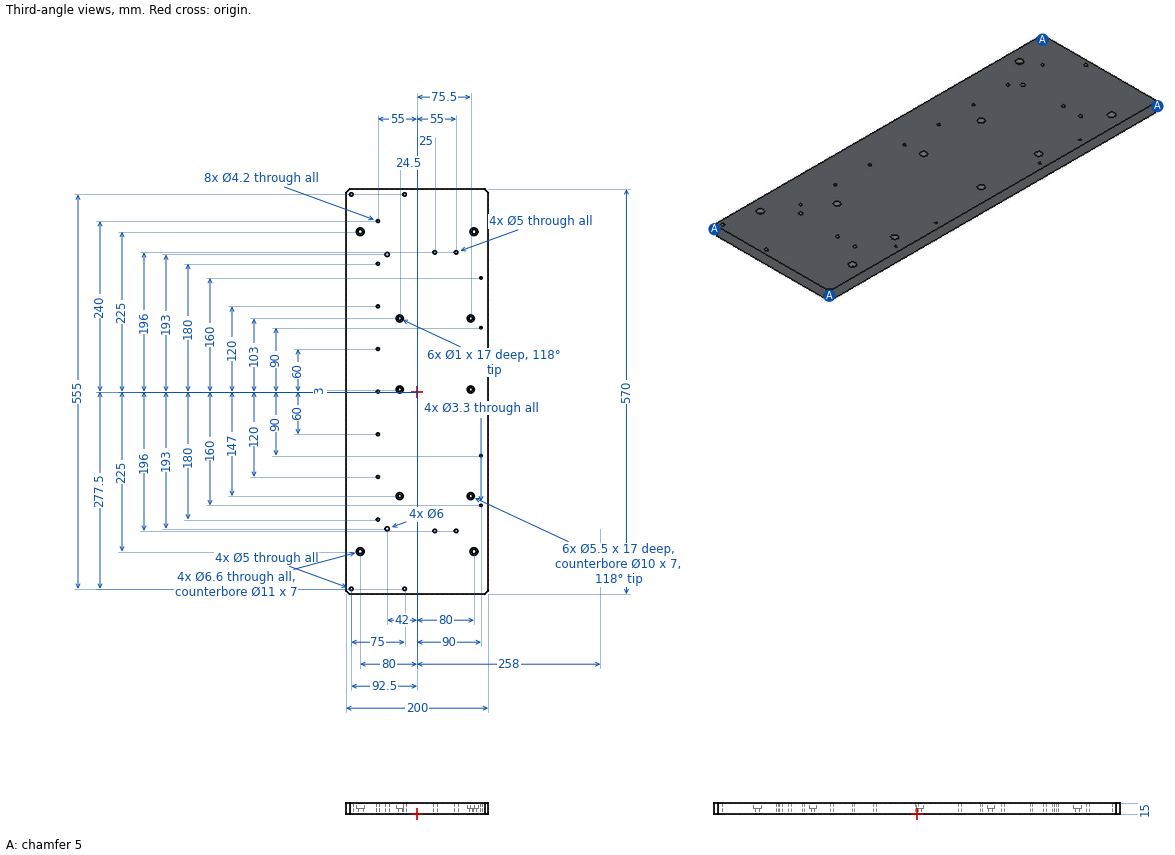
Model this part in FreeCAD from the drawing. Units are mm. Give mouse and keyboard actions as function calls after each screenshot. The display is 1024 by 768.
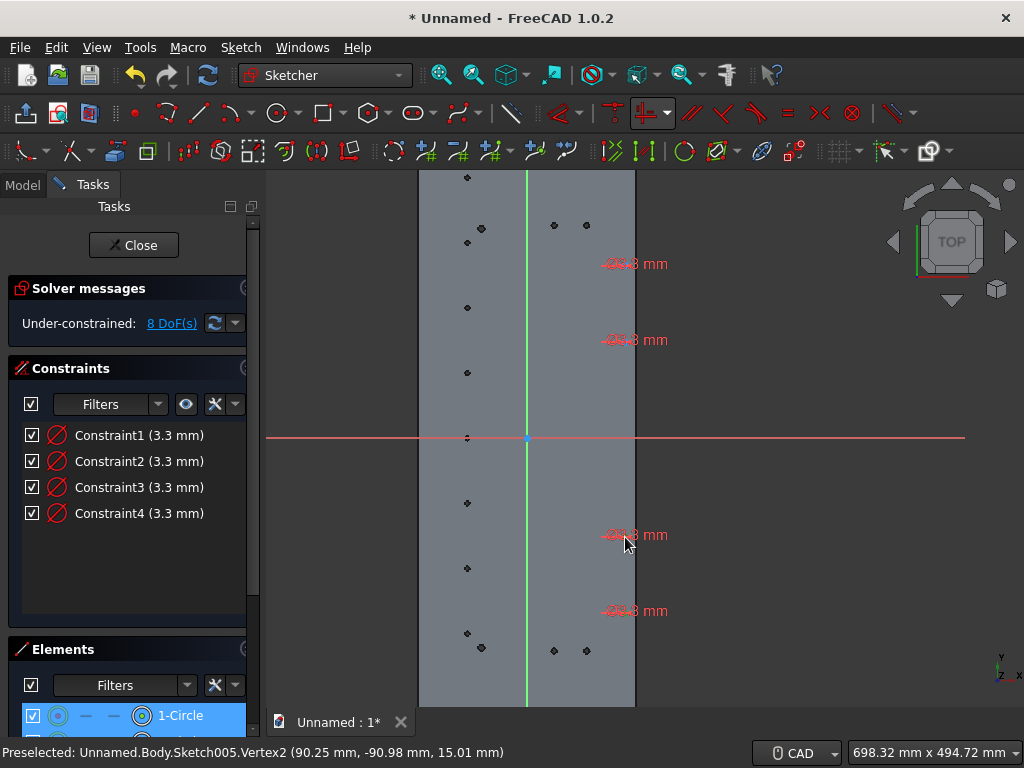
key(v)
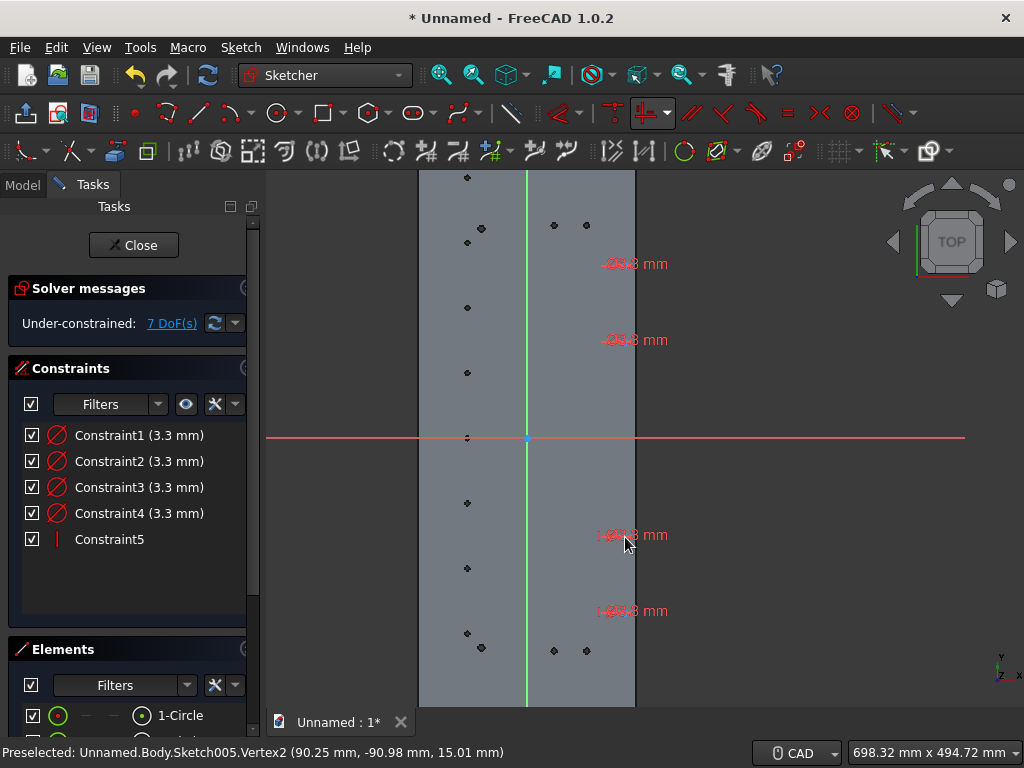
click(625, 537)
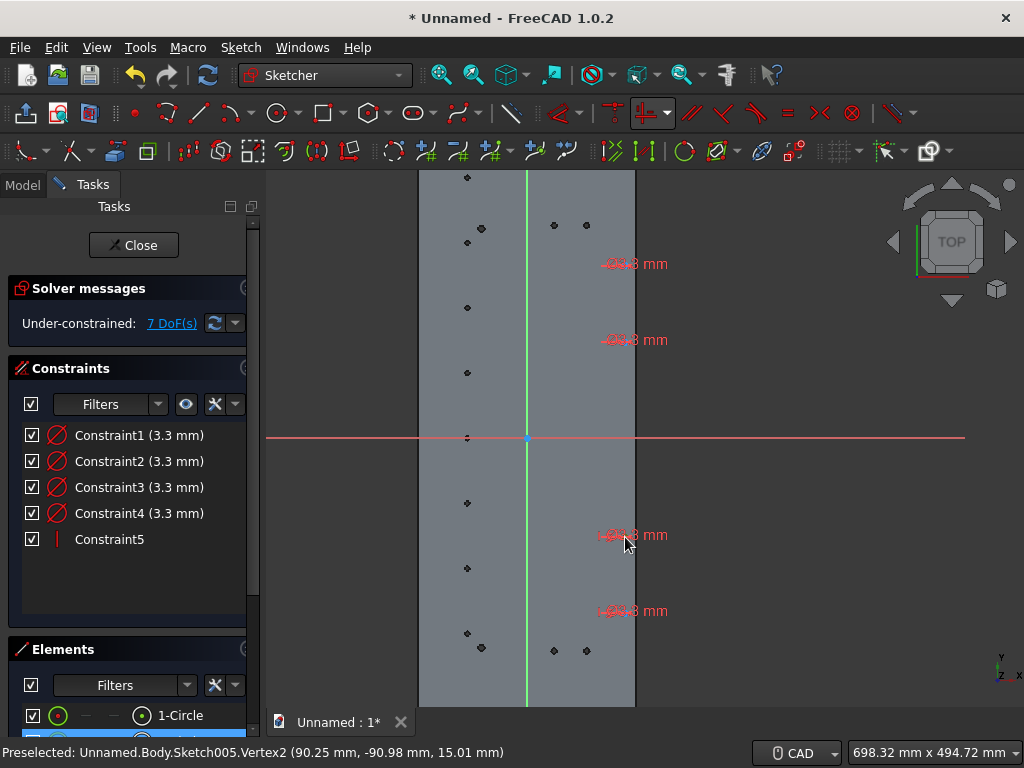
click(625, 342)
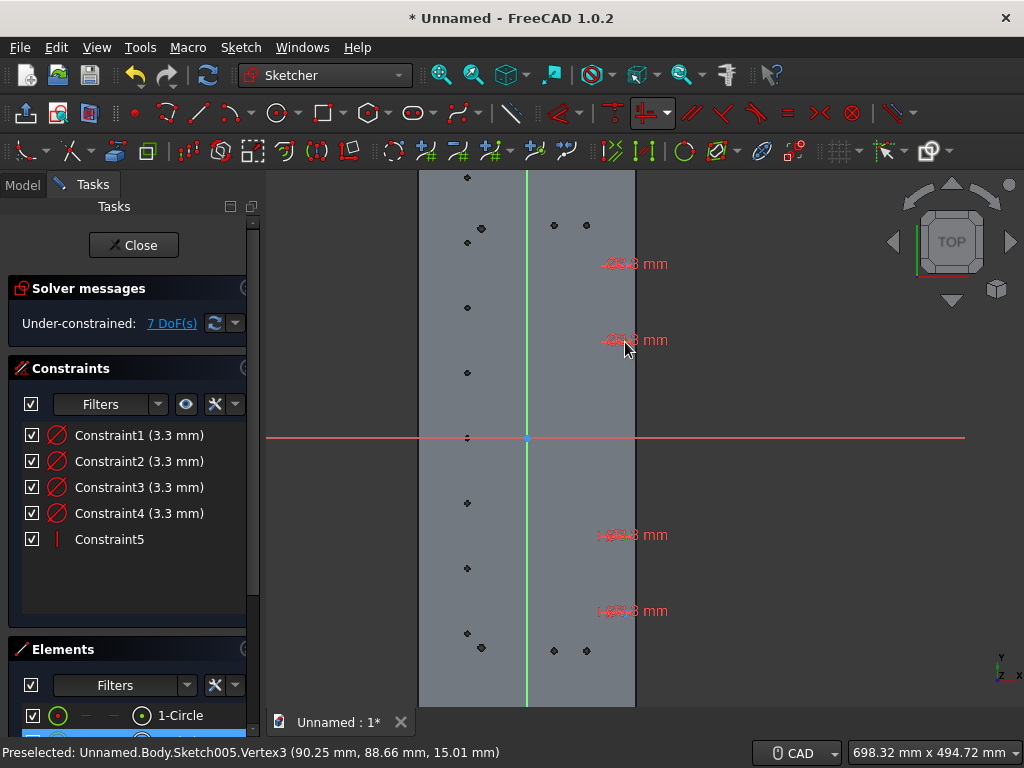
click(670, 114)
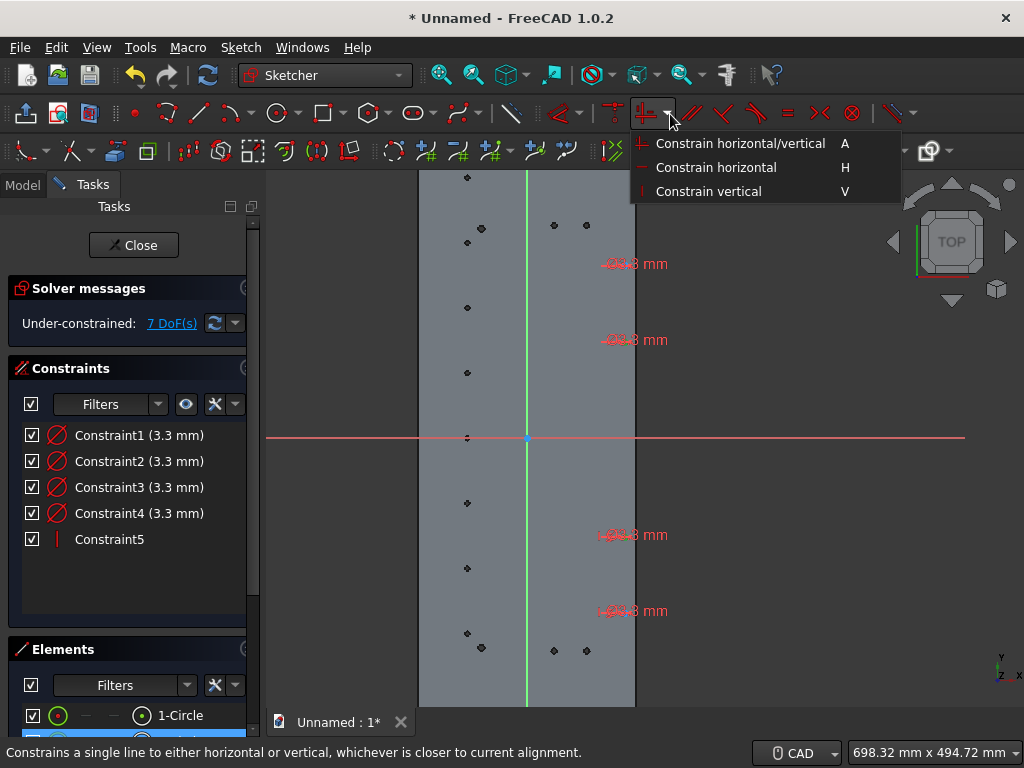
click(766, 191)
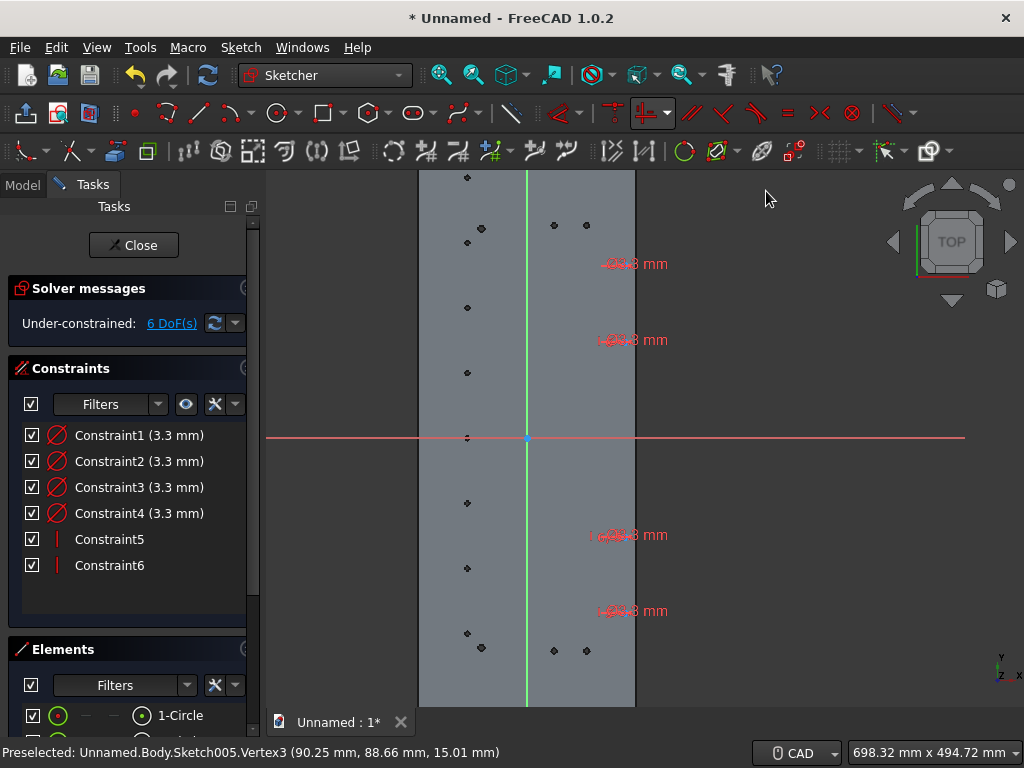
click(625, 342)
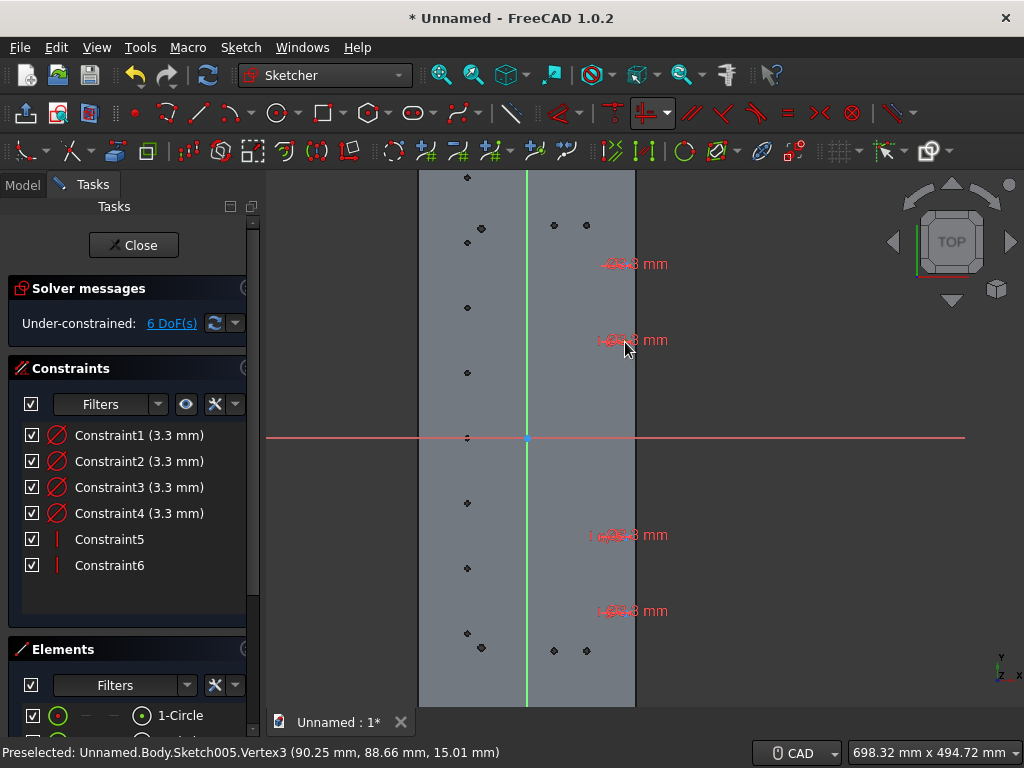
click(625, 266)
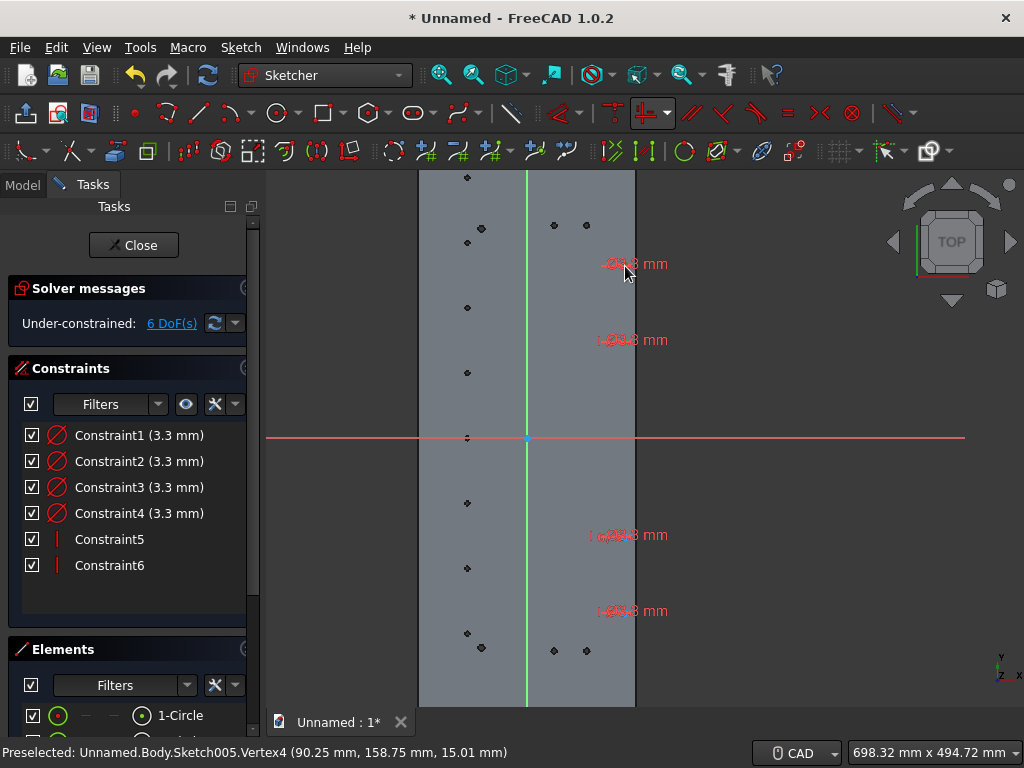
click(670, 114)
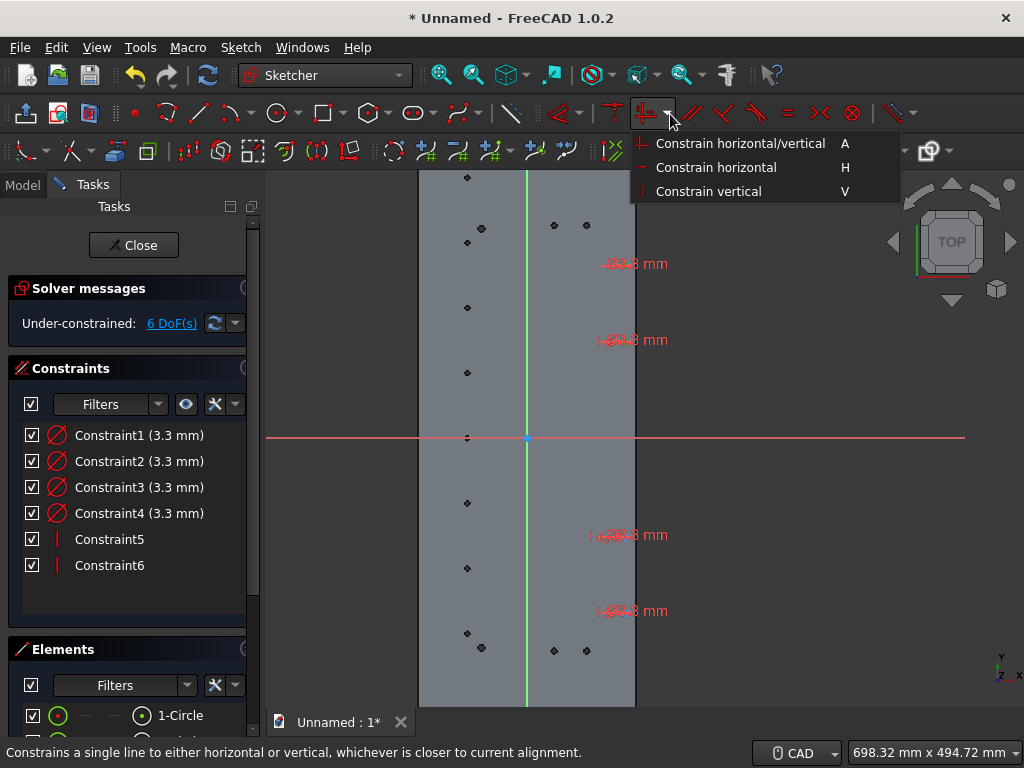
click(766, 191)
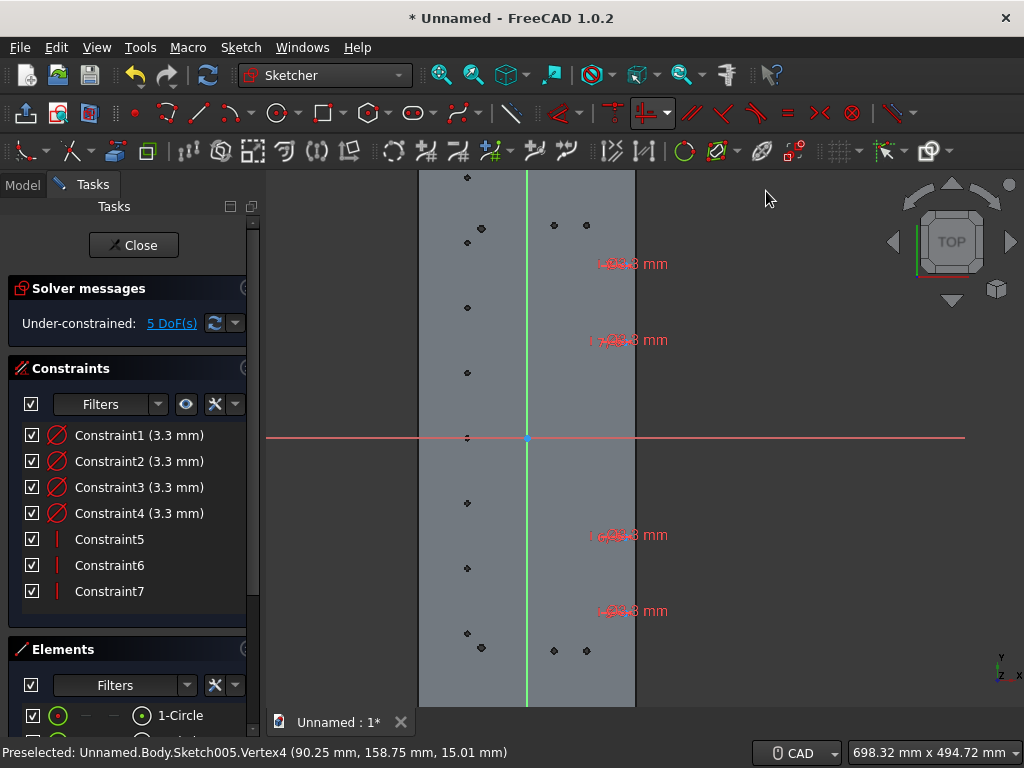
click(558, 114)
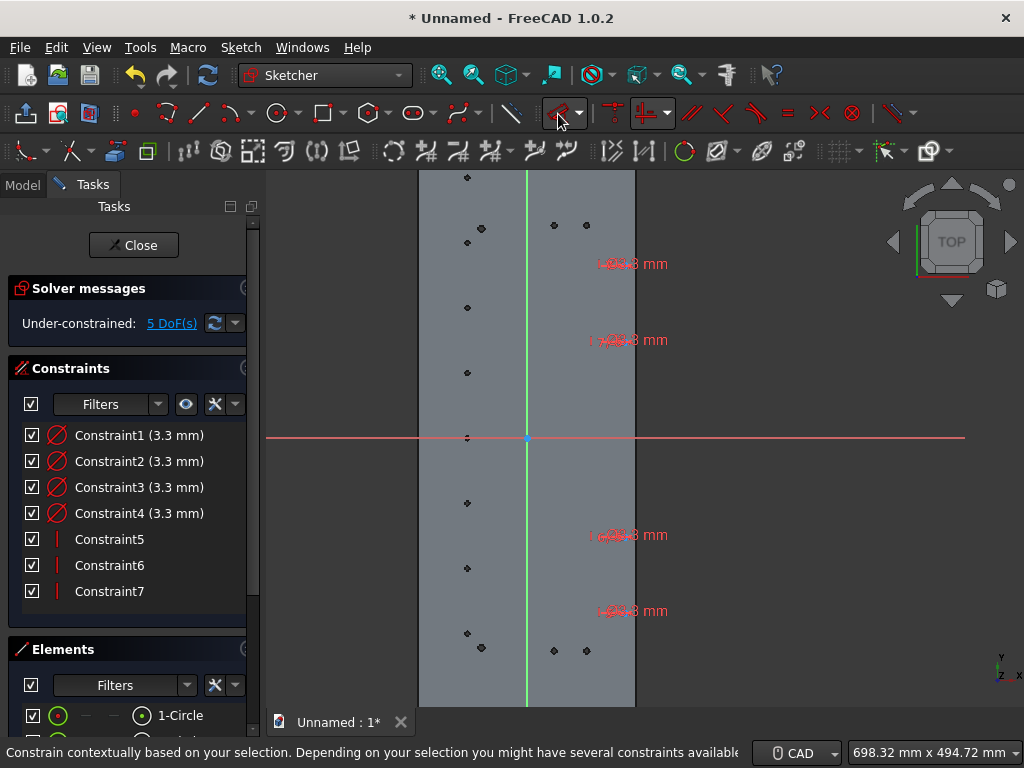
click(625, 613)
click(576, 647)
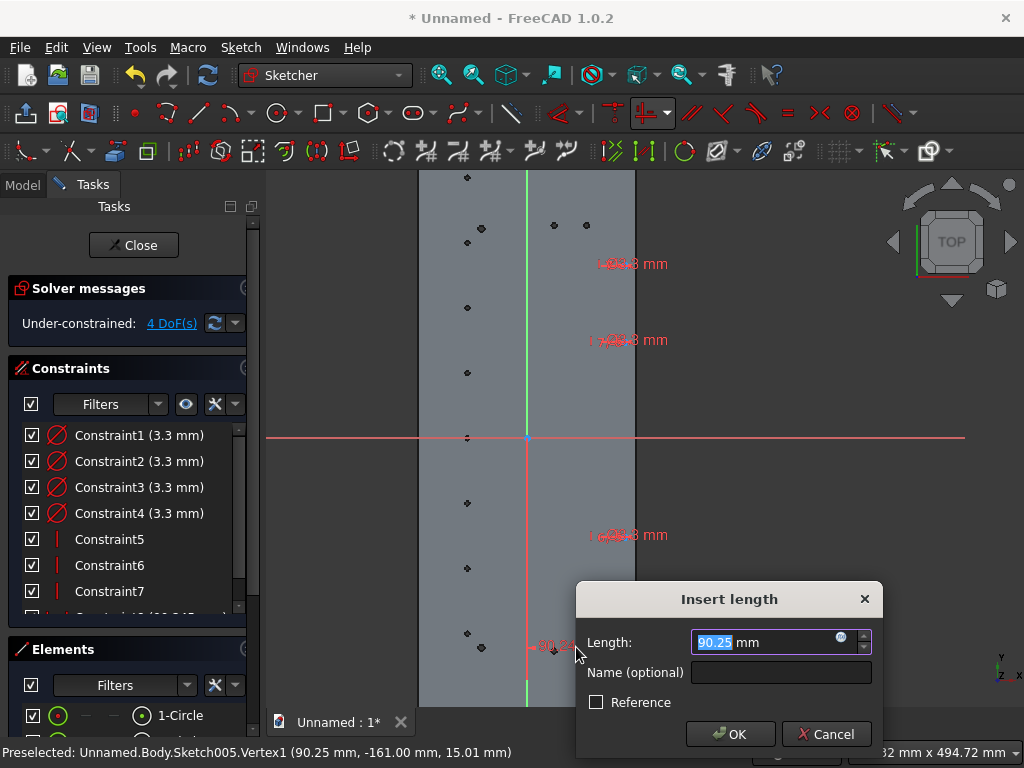
text(90)
key(Return)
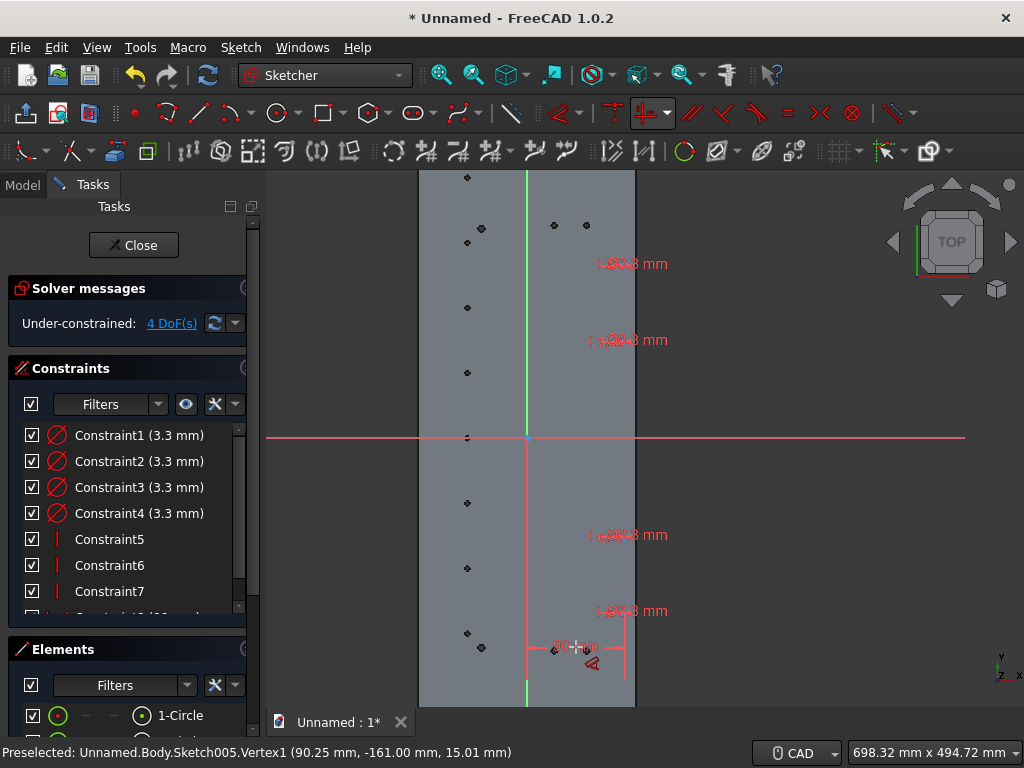
click(625, 537)
click(493, 488)